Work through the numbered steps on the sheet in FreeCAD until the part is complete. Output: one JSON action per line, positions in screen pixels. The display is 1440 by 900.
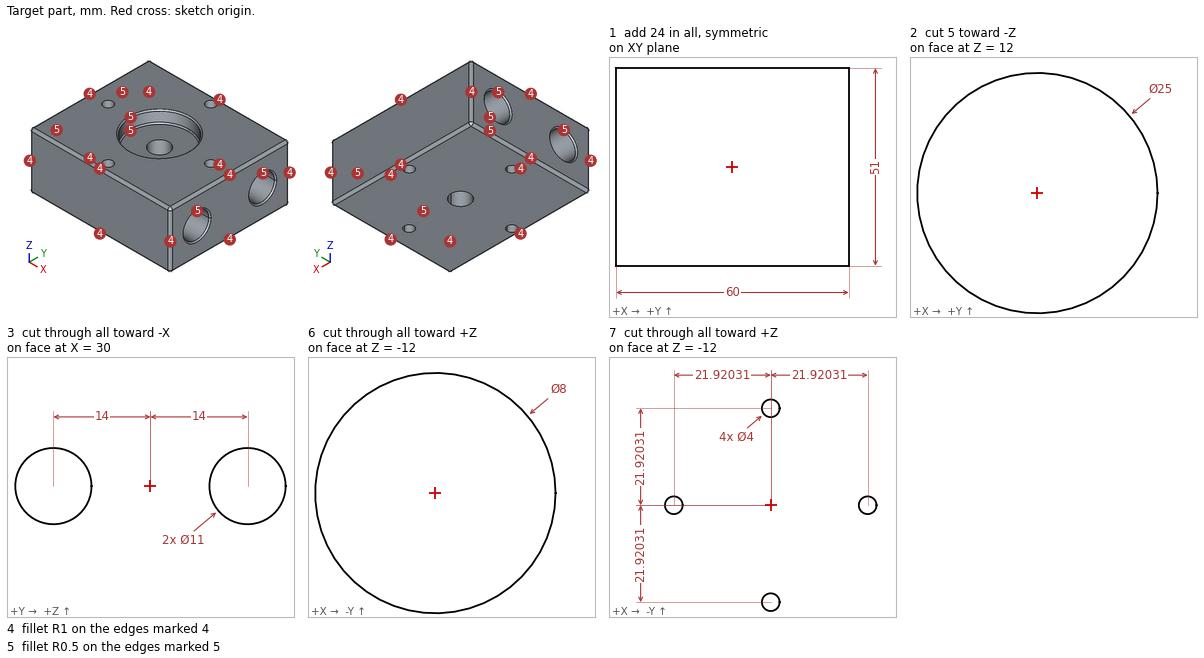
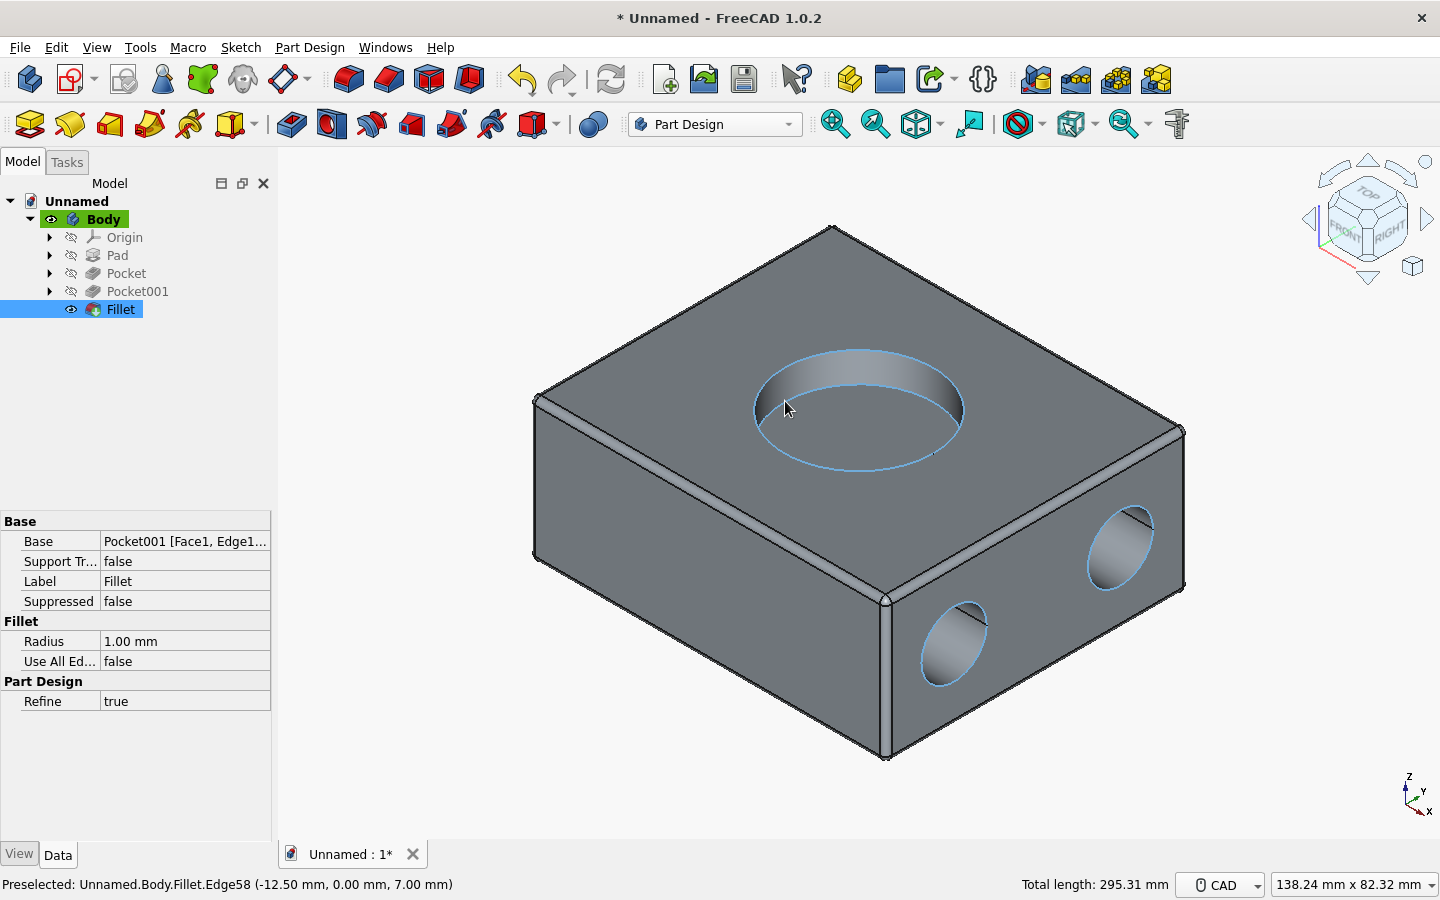
{"action": "left_click", "coordinate": [350, 80]}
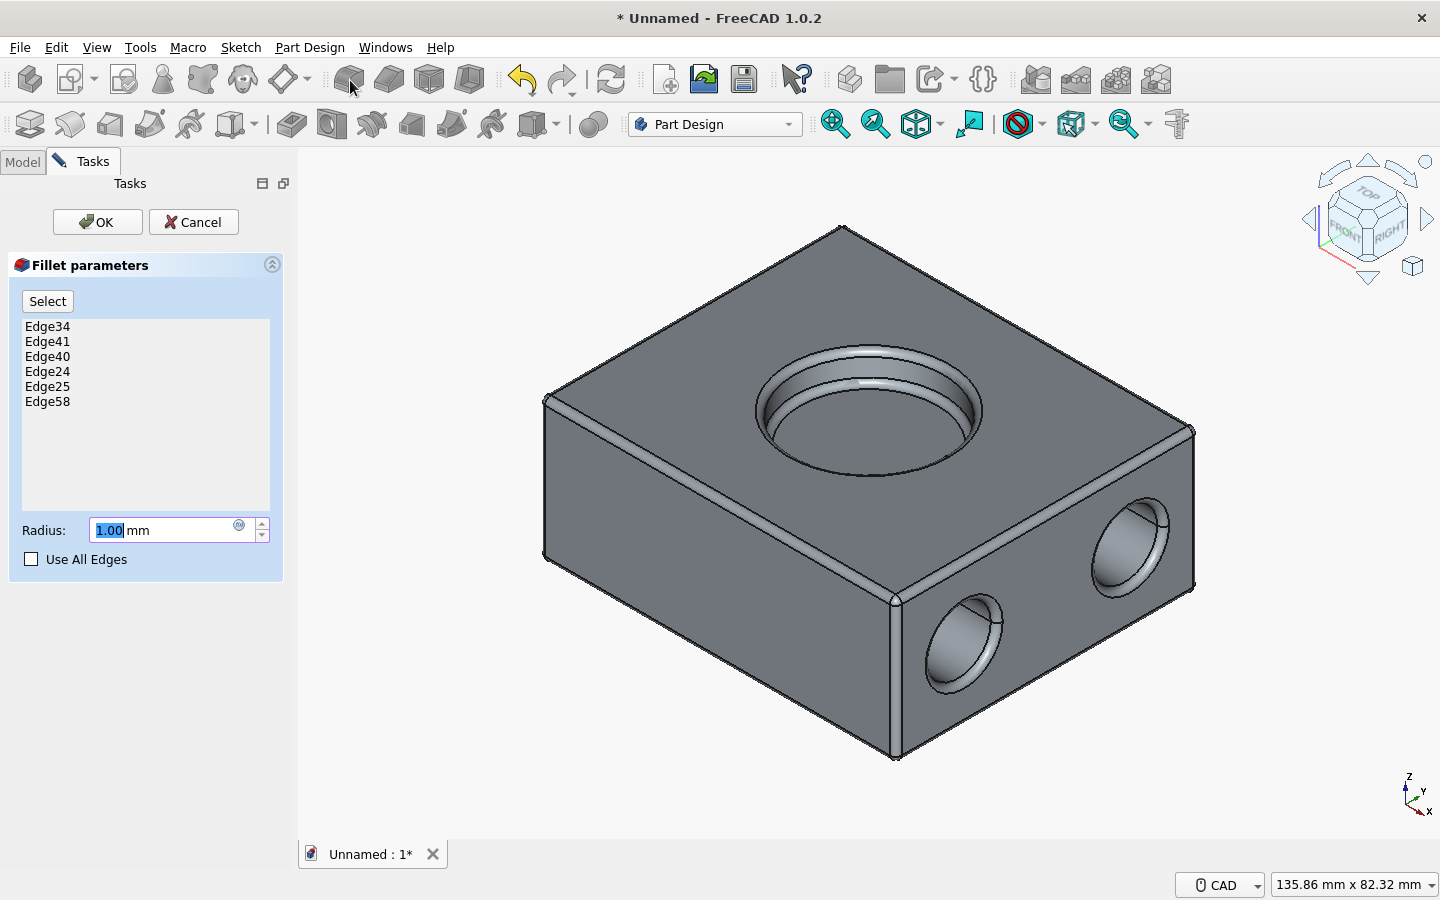
{"action": "type", "text": "0.5"}
{"action": "key", "text": "Tab"}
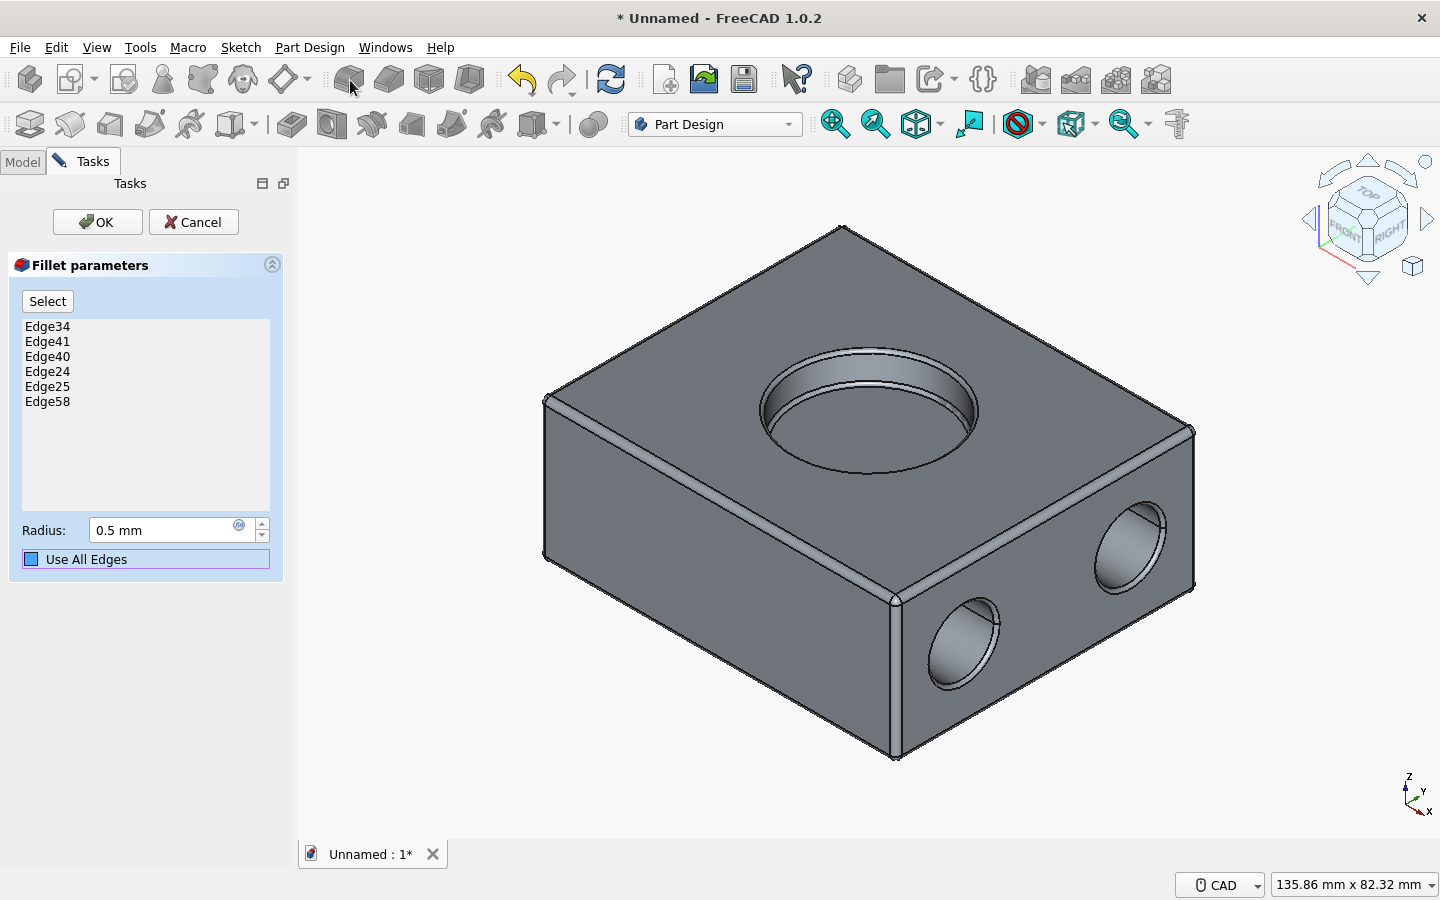
{"action": "left_click", "coordinate": [98, 222]}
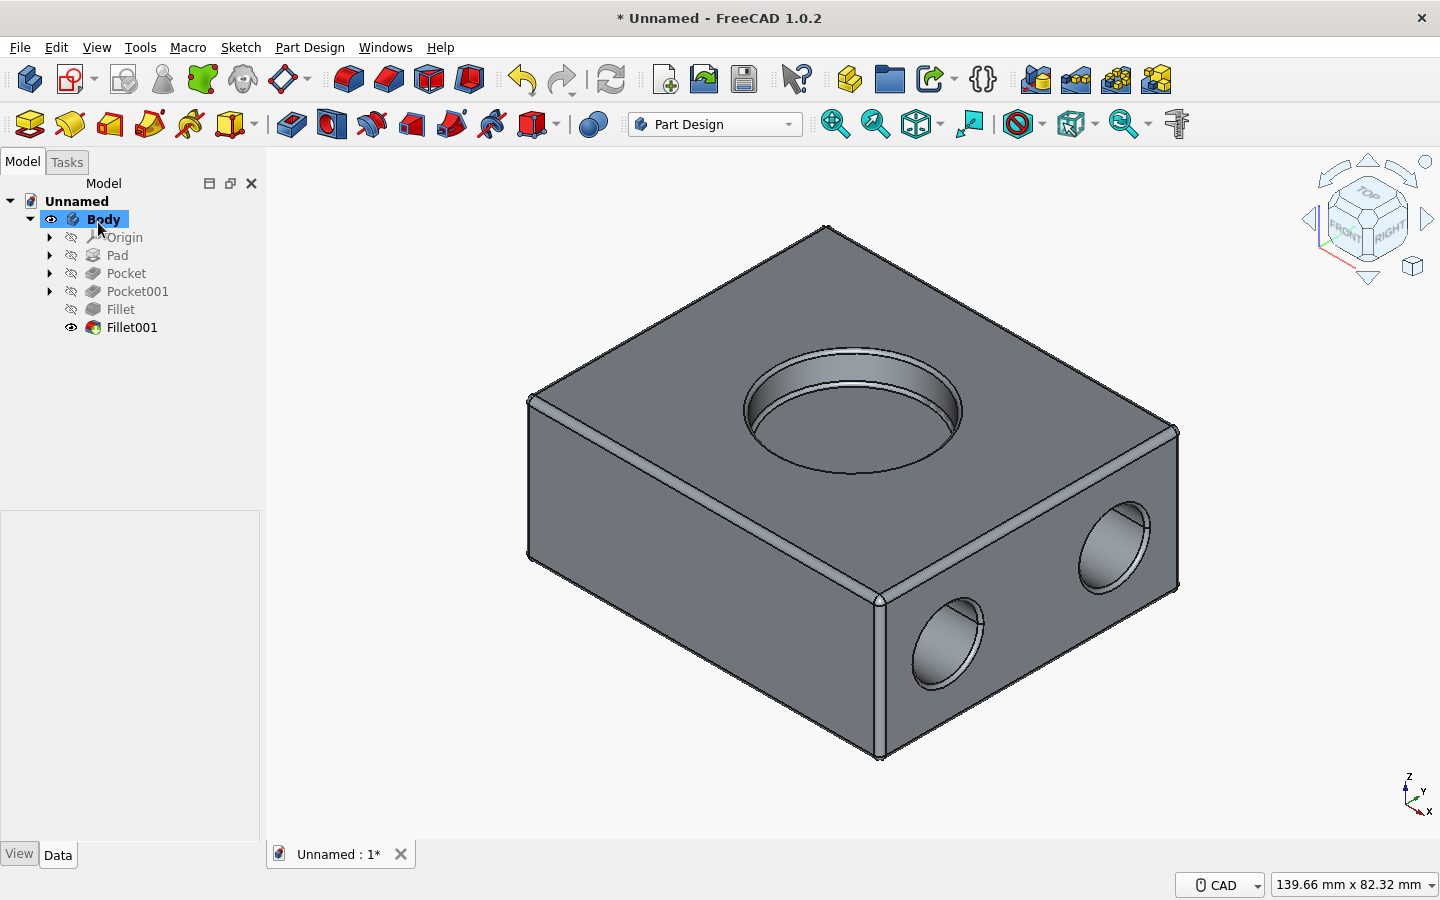
{"action": "key", "text": "5"}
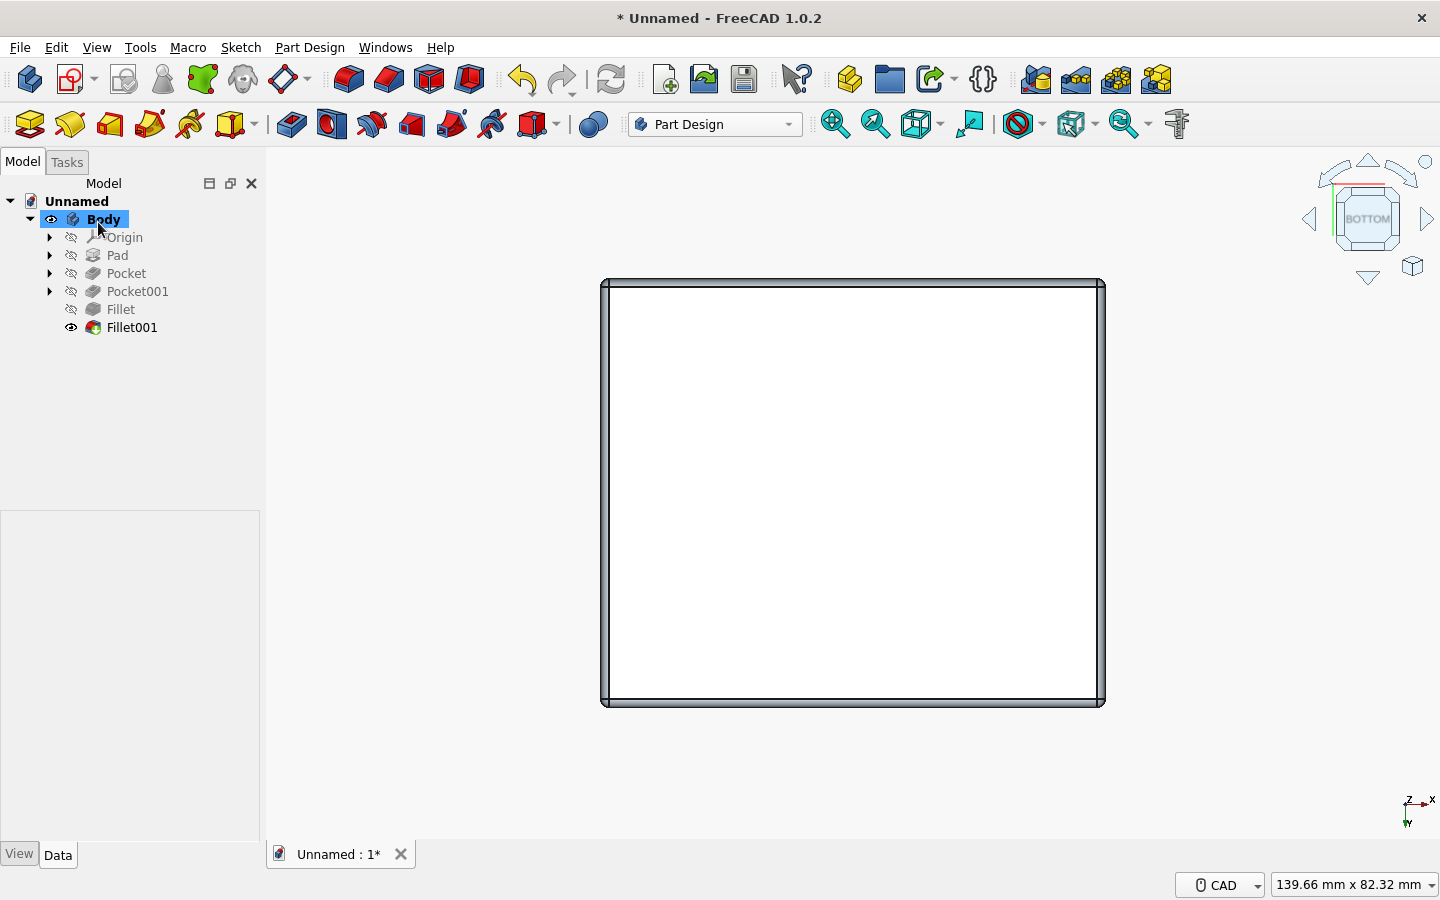
{"action": "left_click", "coordinate": [853, 492]}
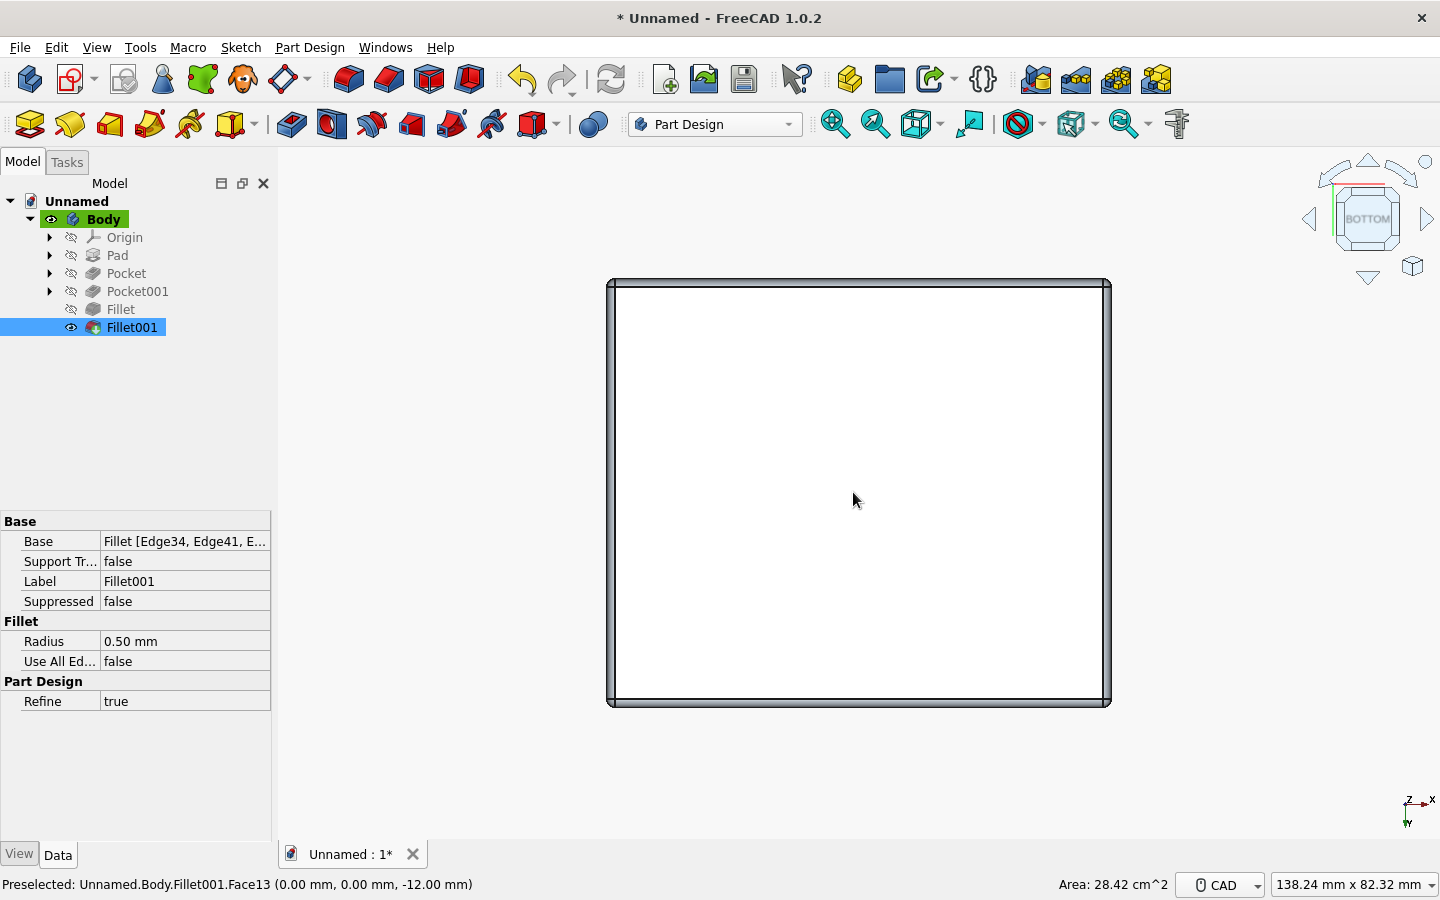
{"action": "left_click", "coordinate": [70, 80]}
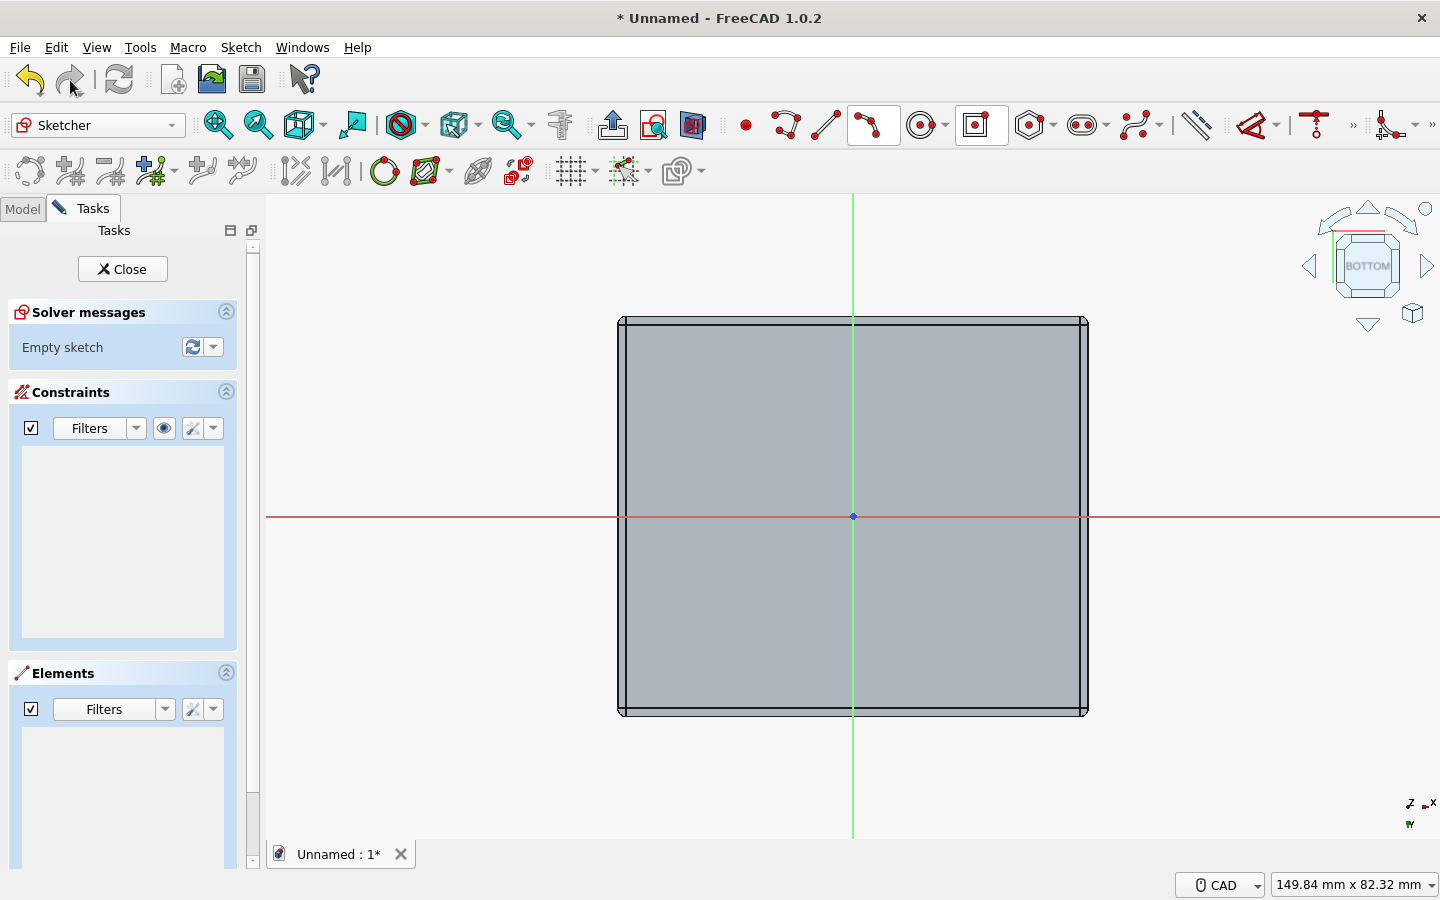
{"action": "scroll", "coordinate": [867, 516], "scroll_direction": "up", "scroll_amount": 9}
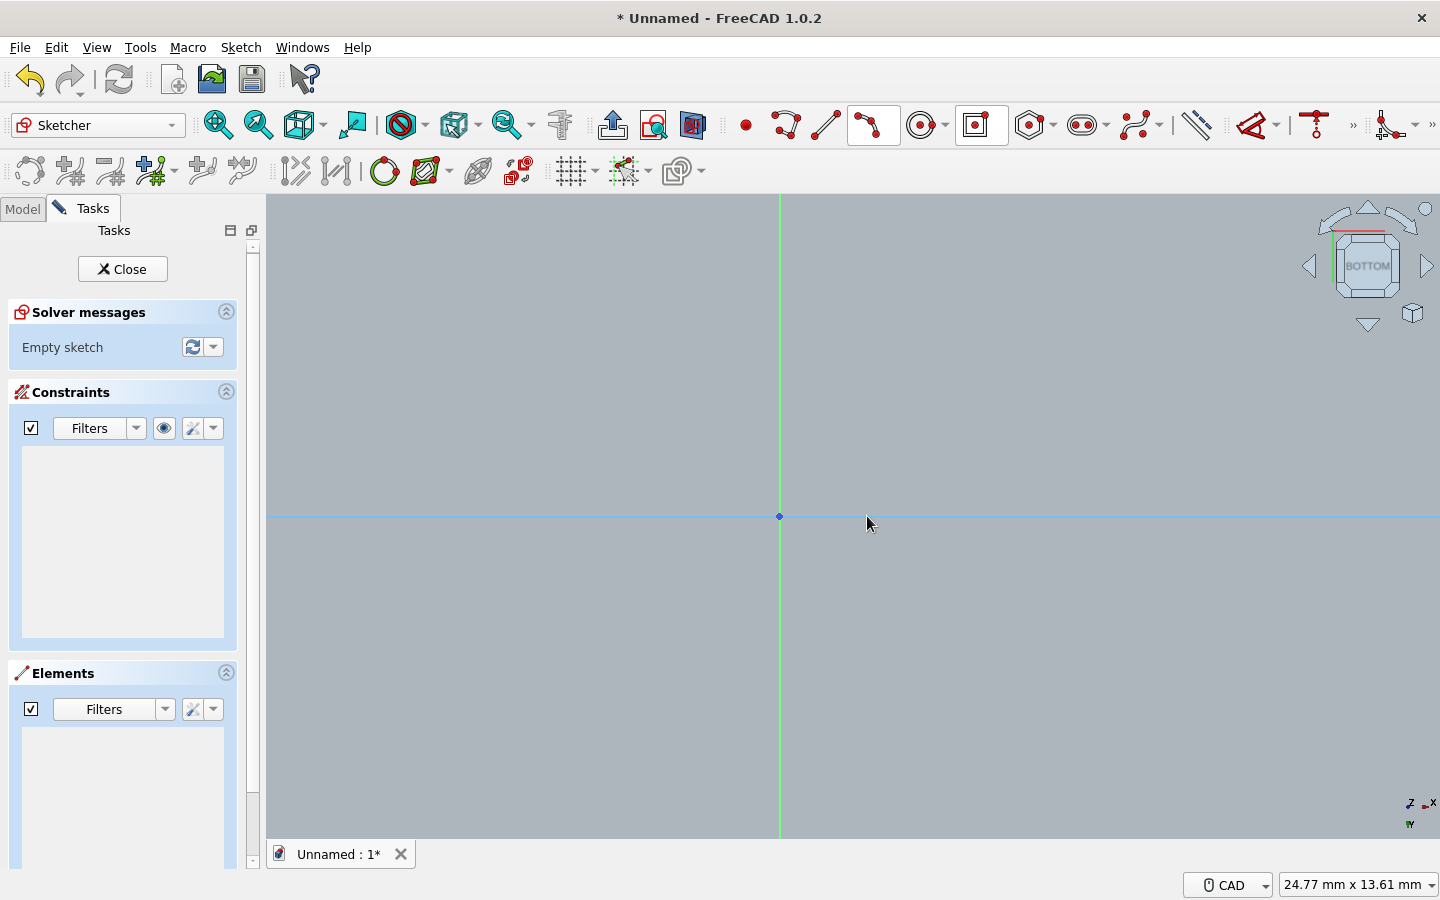
{"action": "left_click", "coordinate": [922, 126]}